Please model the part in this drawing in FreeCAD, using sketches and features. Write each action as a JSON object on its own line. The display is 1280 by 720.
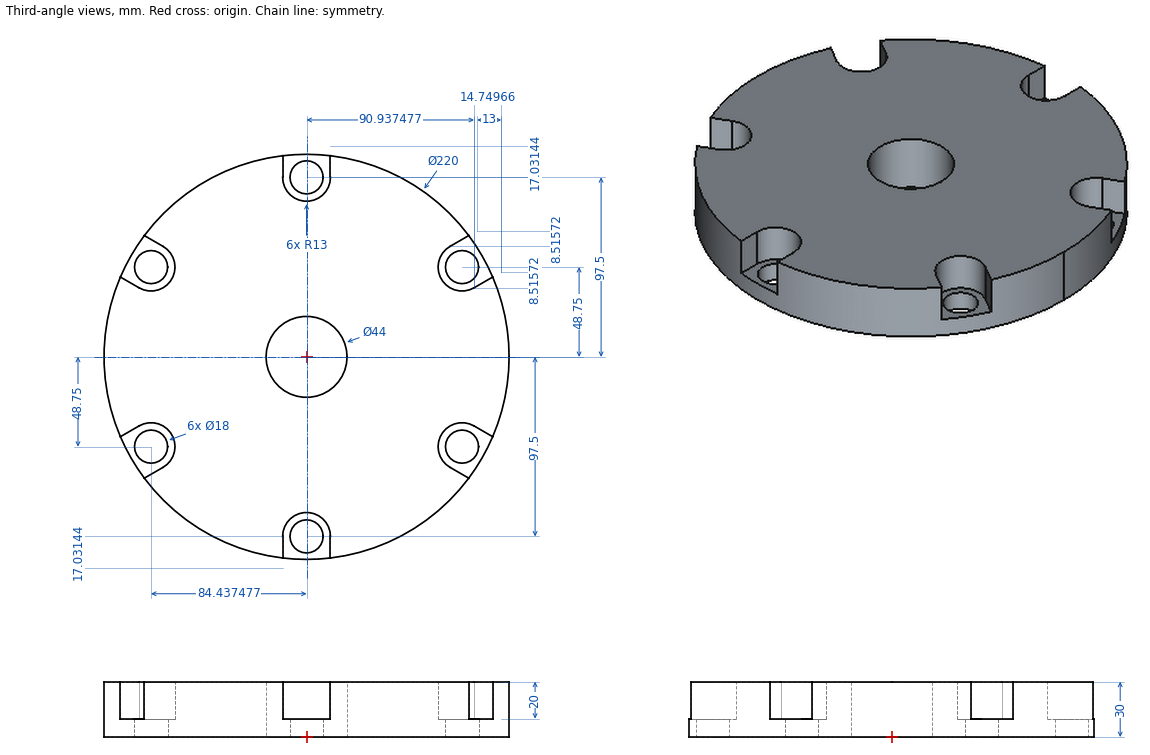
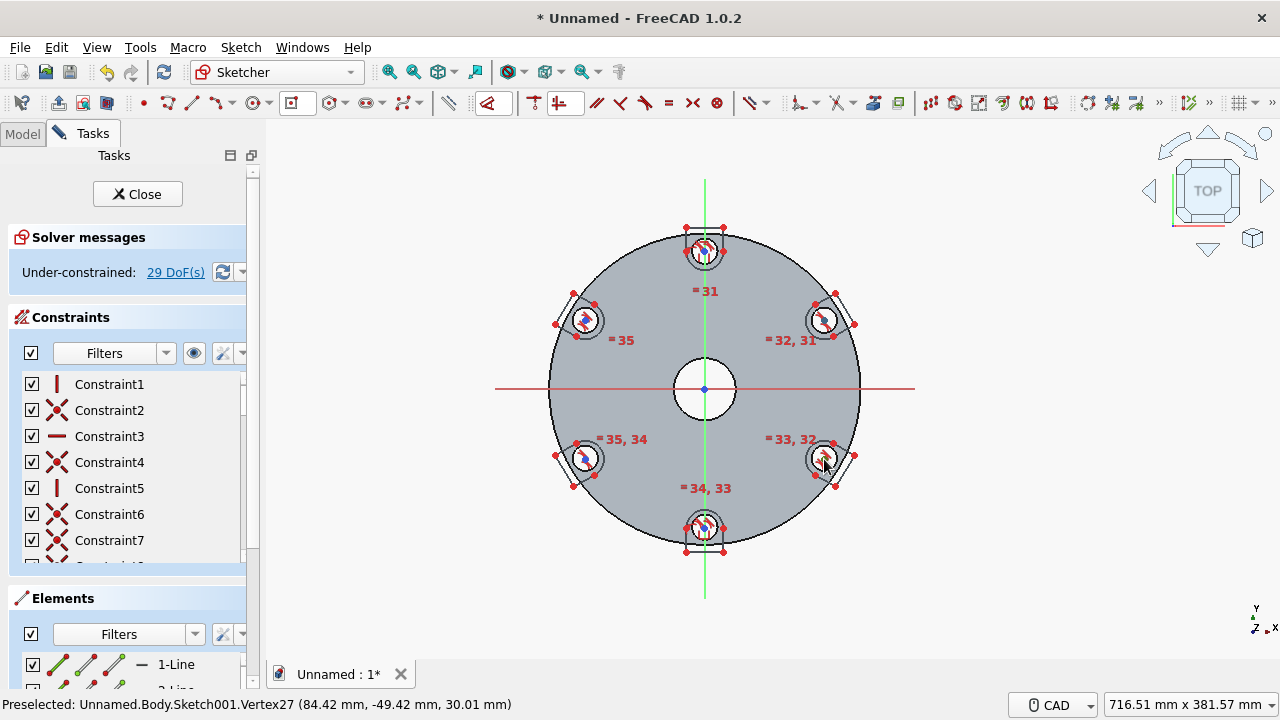
{"action": "left_click", "coordinate": [529, 389]}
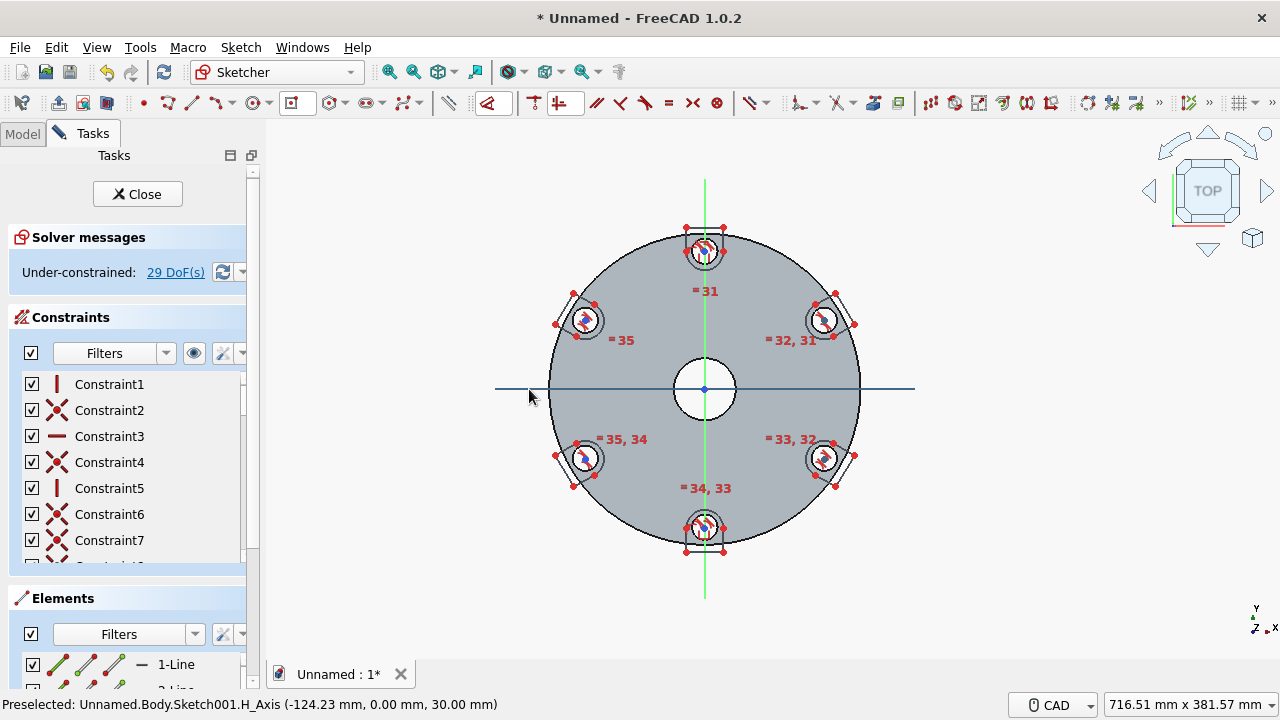
{"action": "key", "text": "s"}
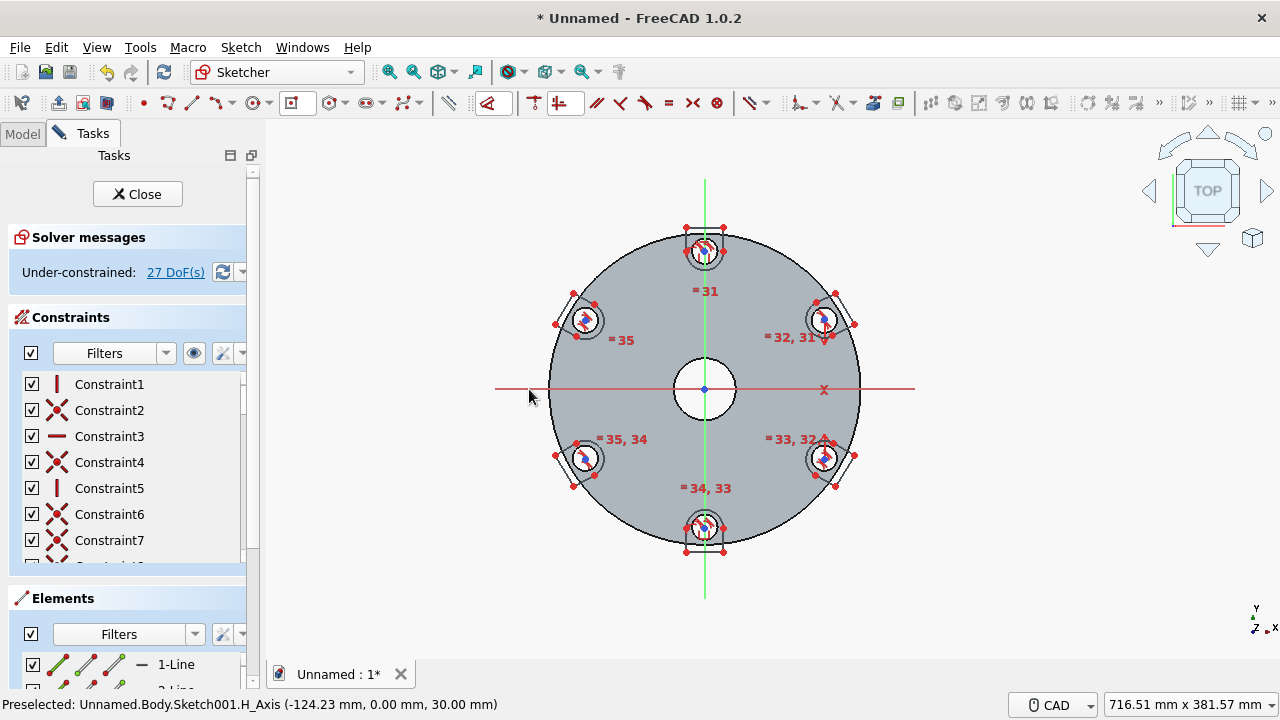
{"action": "left_click", "coordinate": [825, 459]}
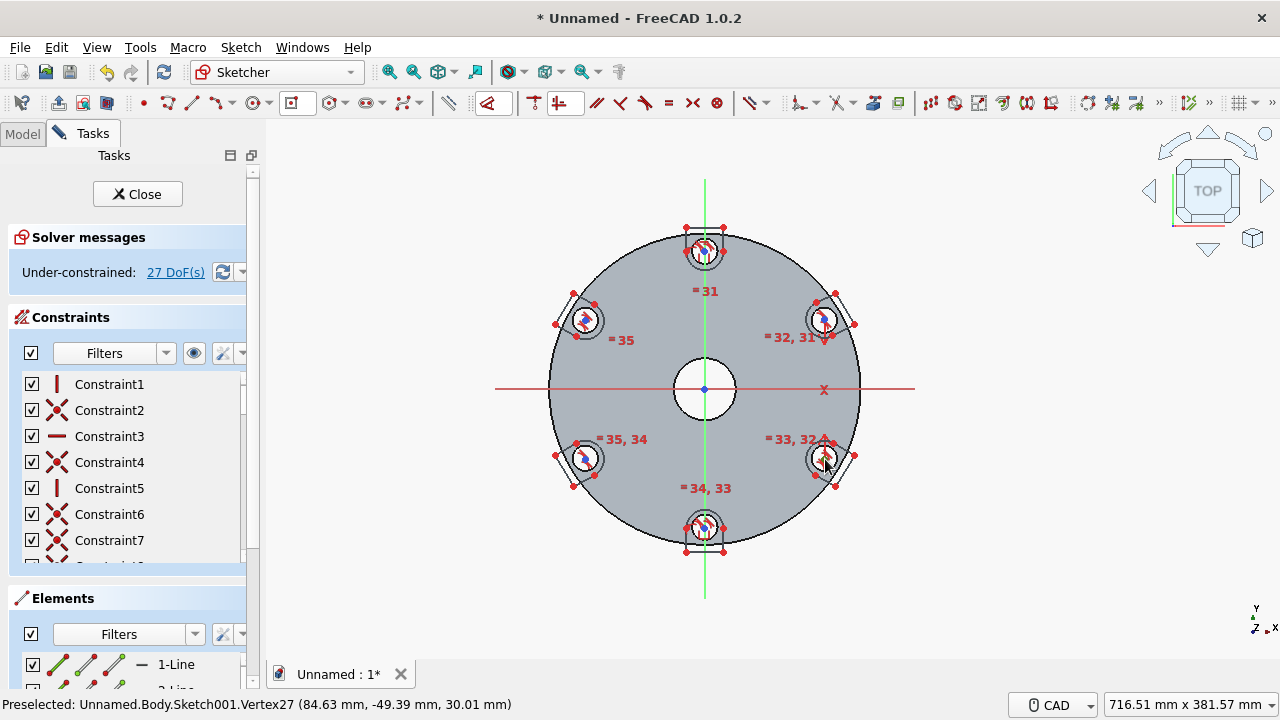
{"action": "left_click", "coordinate": [586, 459]}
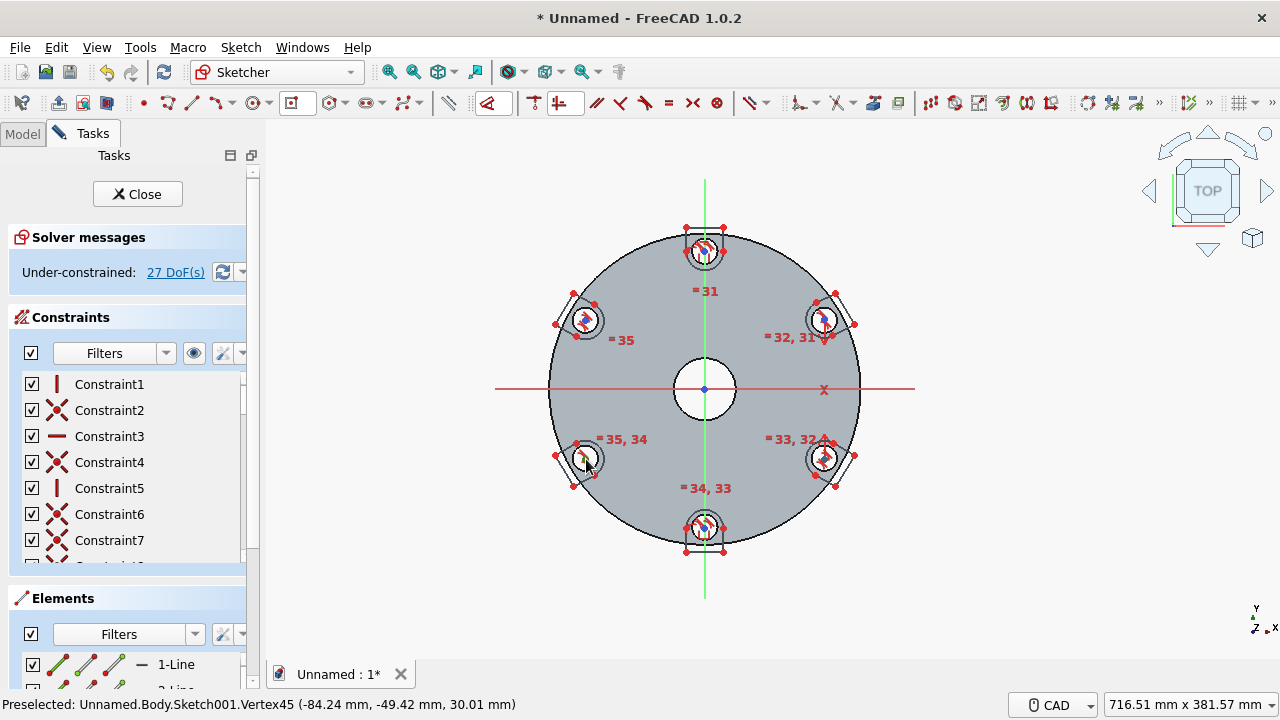
{"action": "left_click", "coordinate": [705, 596]}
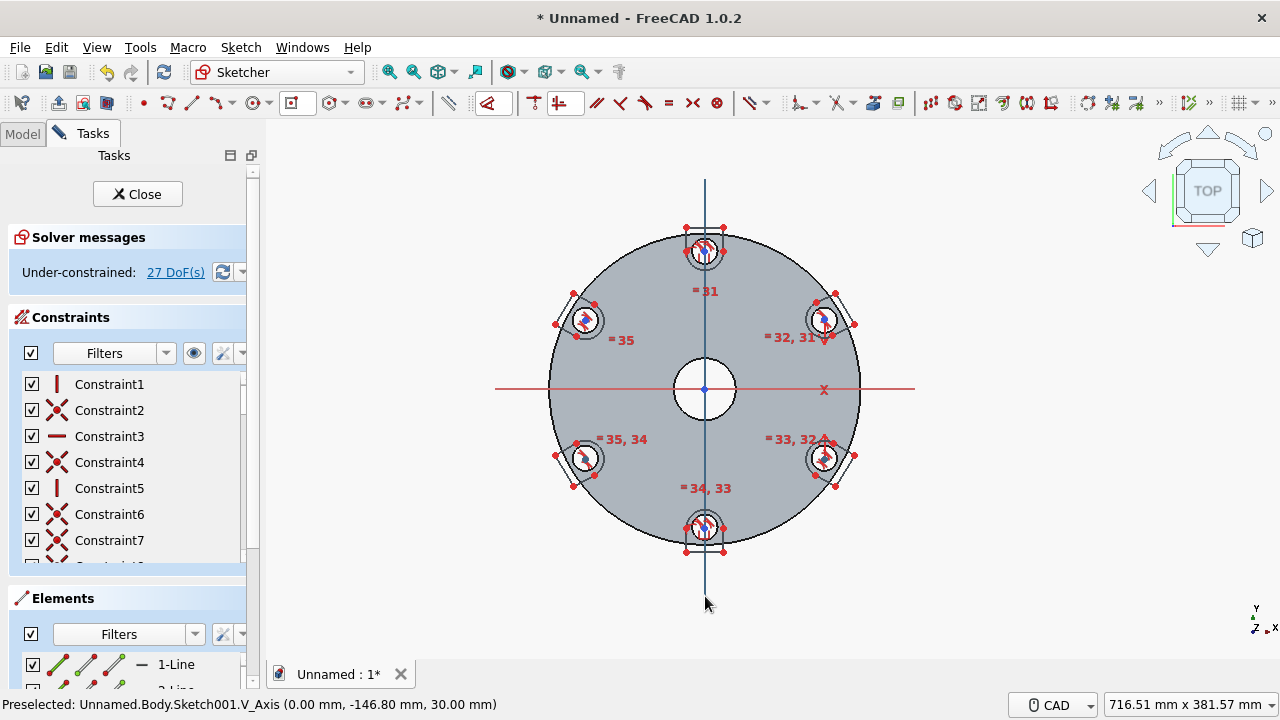
{"action": "key", "text": "s"}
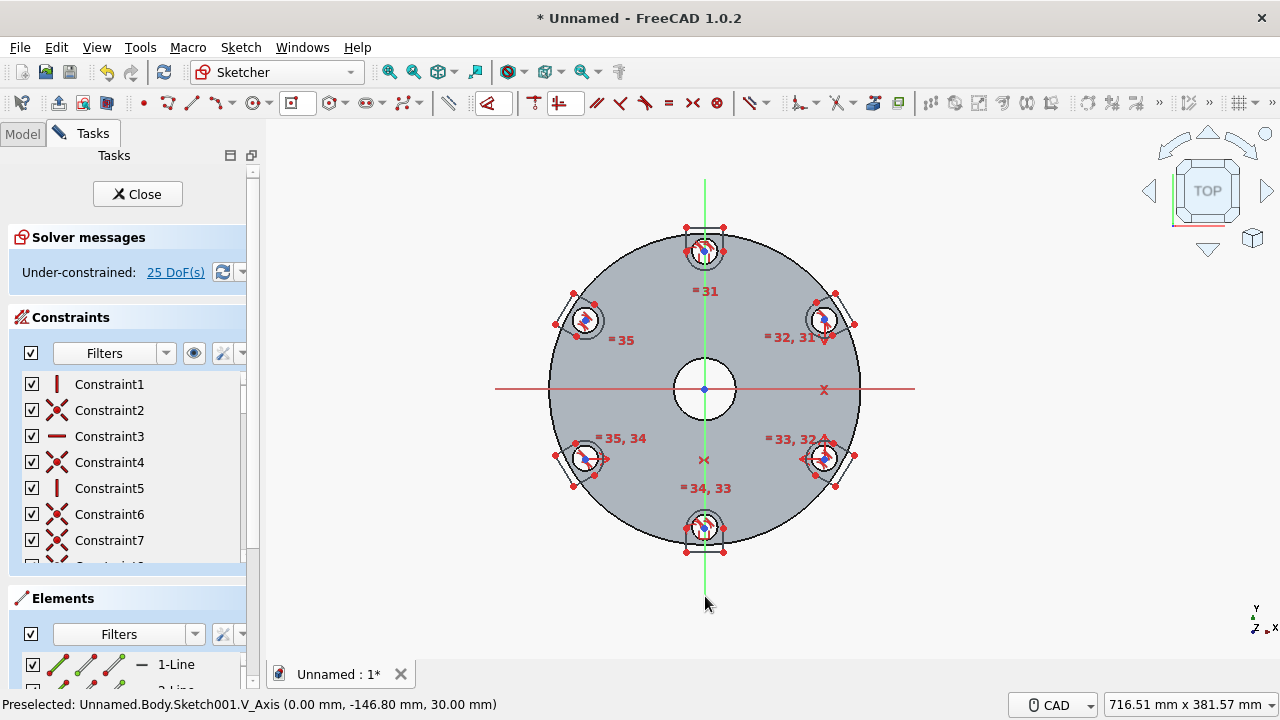
{"action": "left_click", "coordinate": [825, 319]}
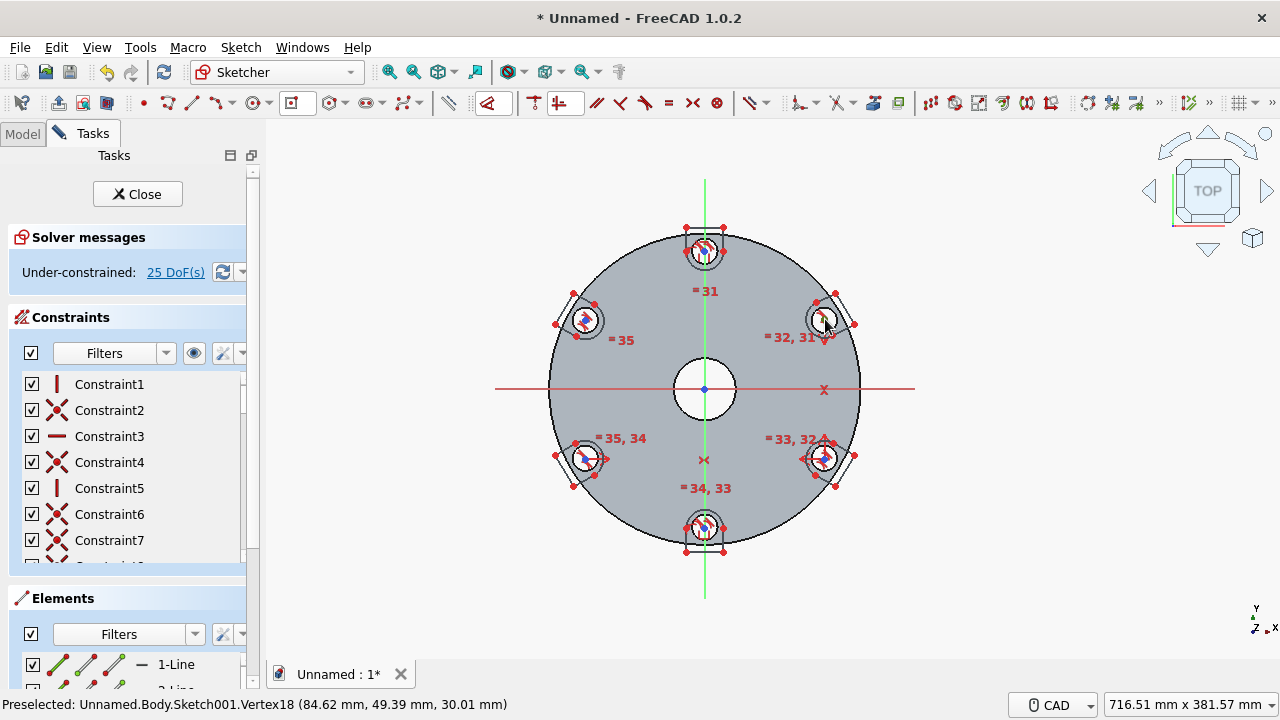
{"action": "left_click", "coordinate": [586, 321]}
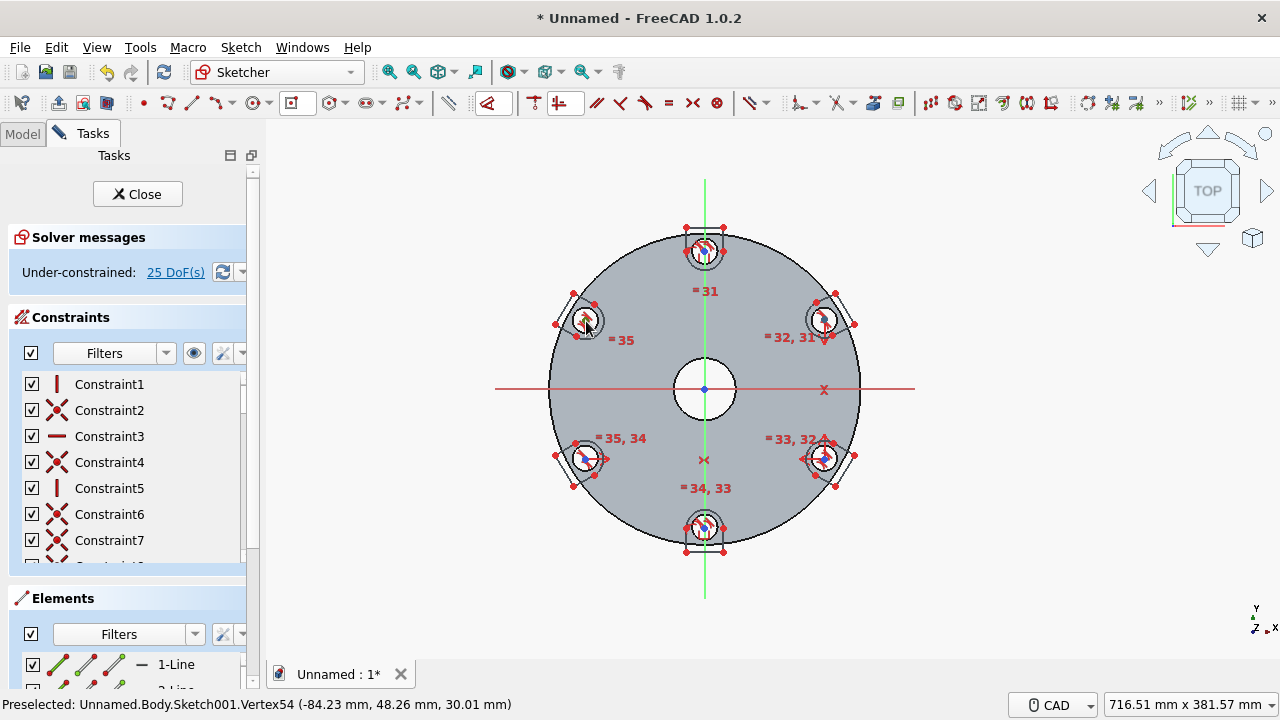
{"action": "left_click", "coordinate": [705, 596]}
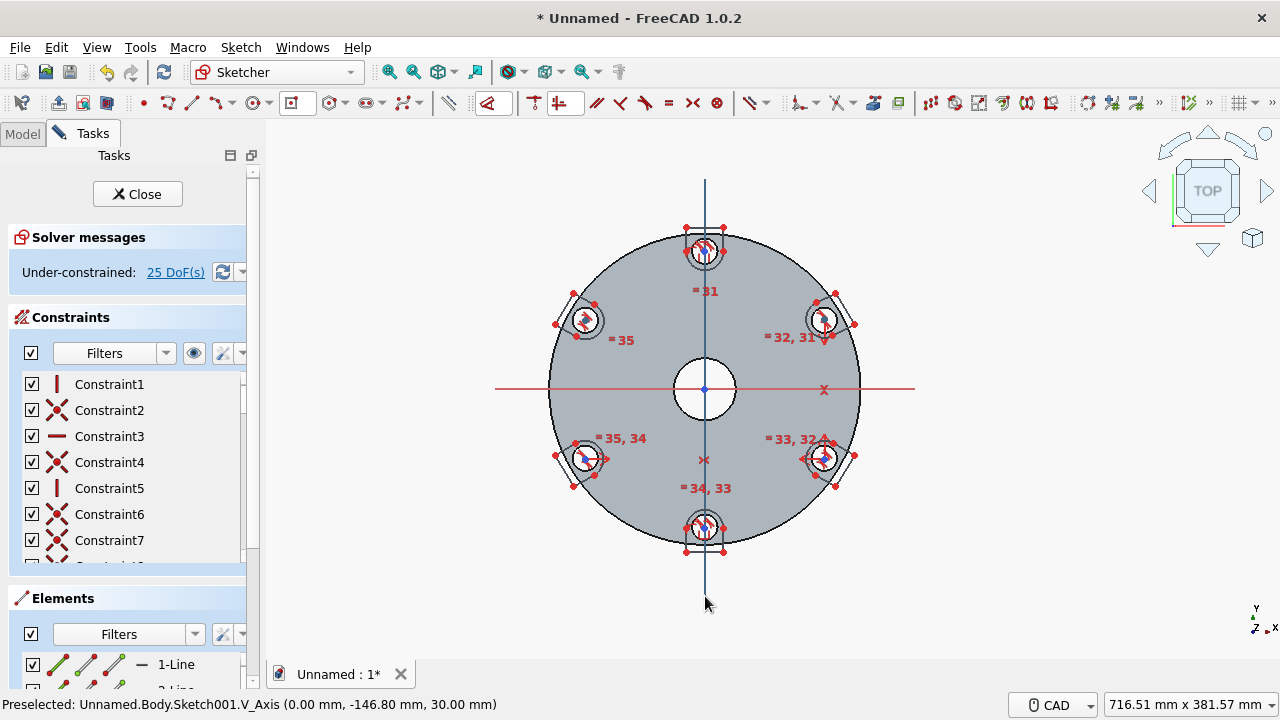
{"action": "left_click", "coordinate": [694, 104]}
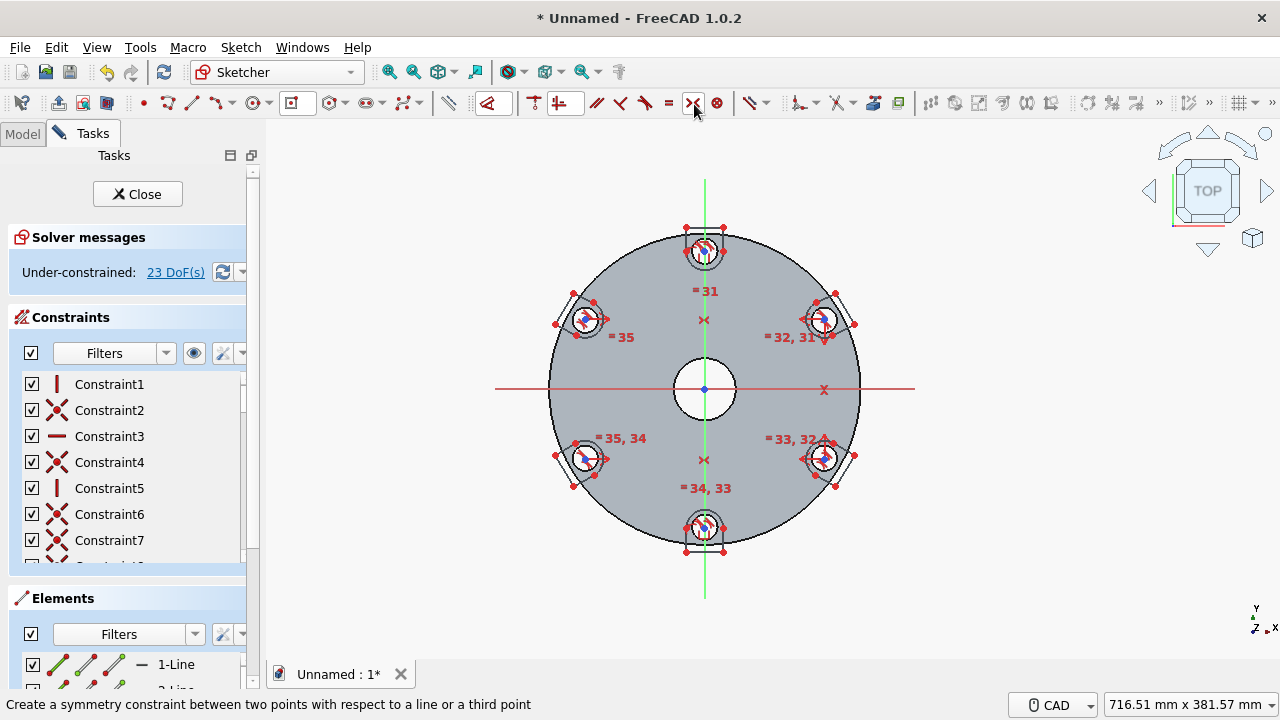
{"action": "left_click", "coordinate": [836, 293]}